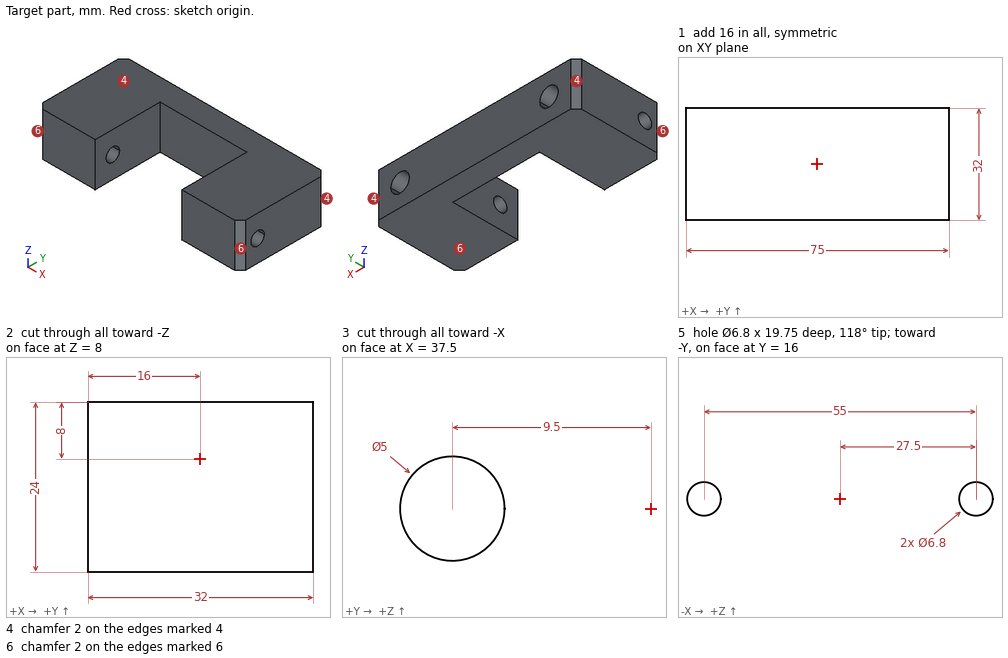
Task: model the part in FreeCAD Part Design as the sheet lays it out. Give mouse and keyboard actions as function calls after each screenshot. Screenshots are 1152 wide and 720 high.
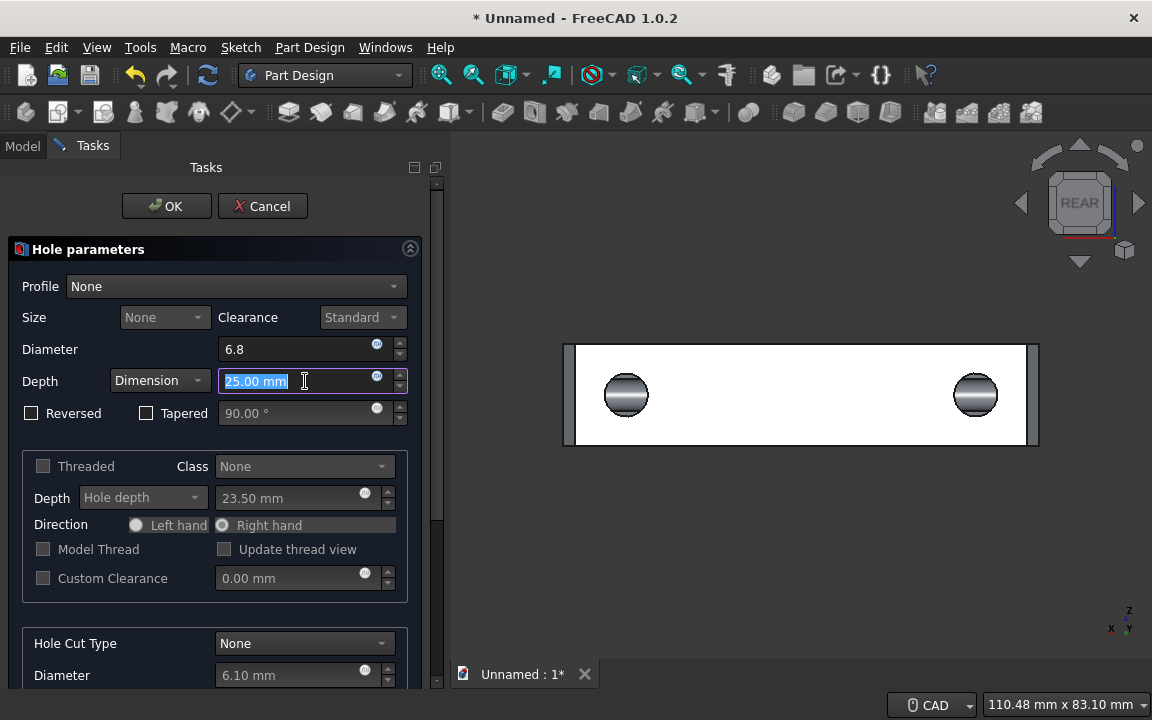
text(19.75)
key(Tab)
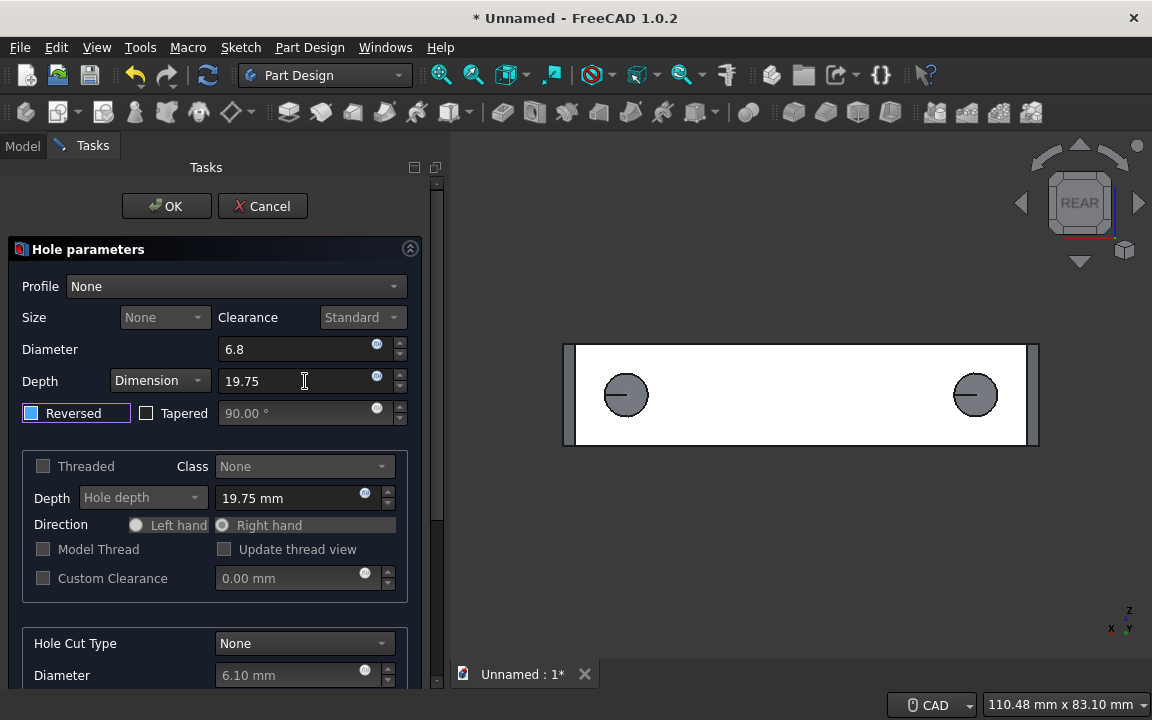
click(167, 206)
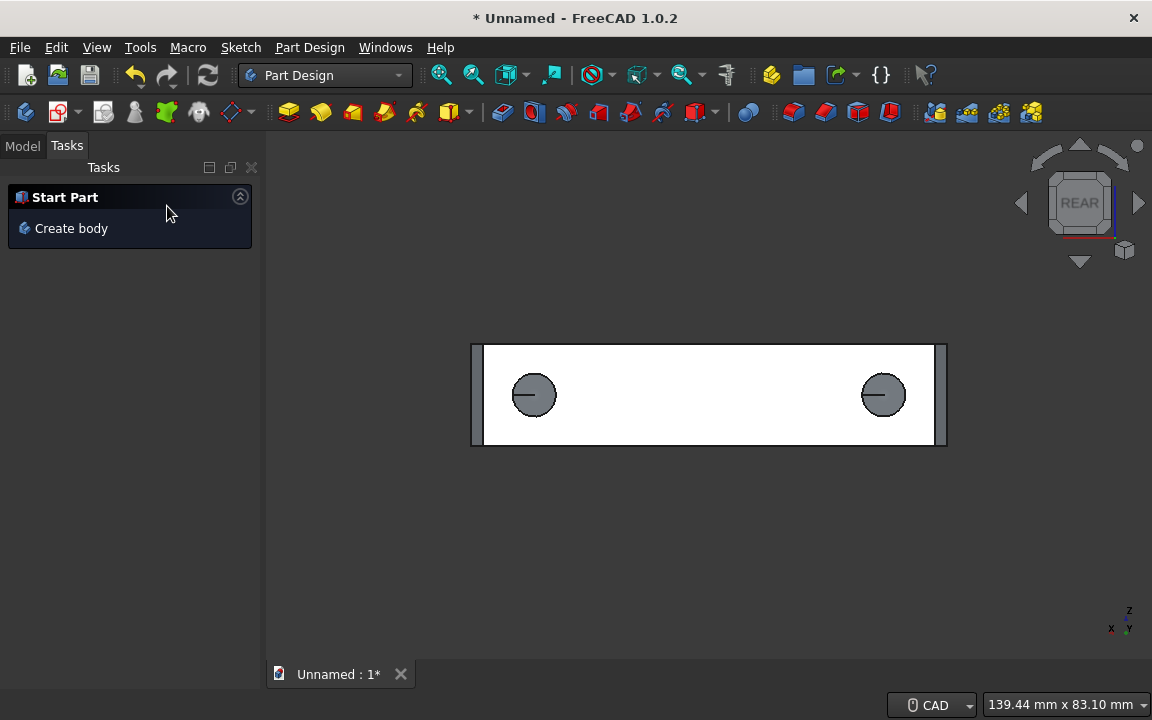
key(0)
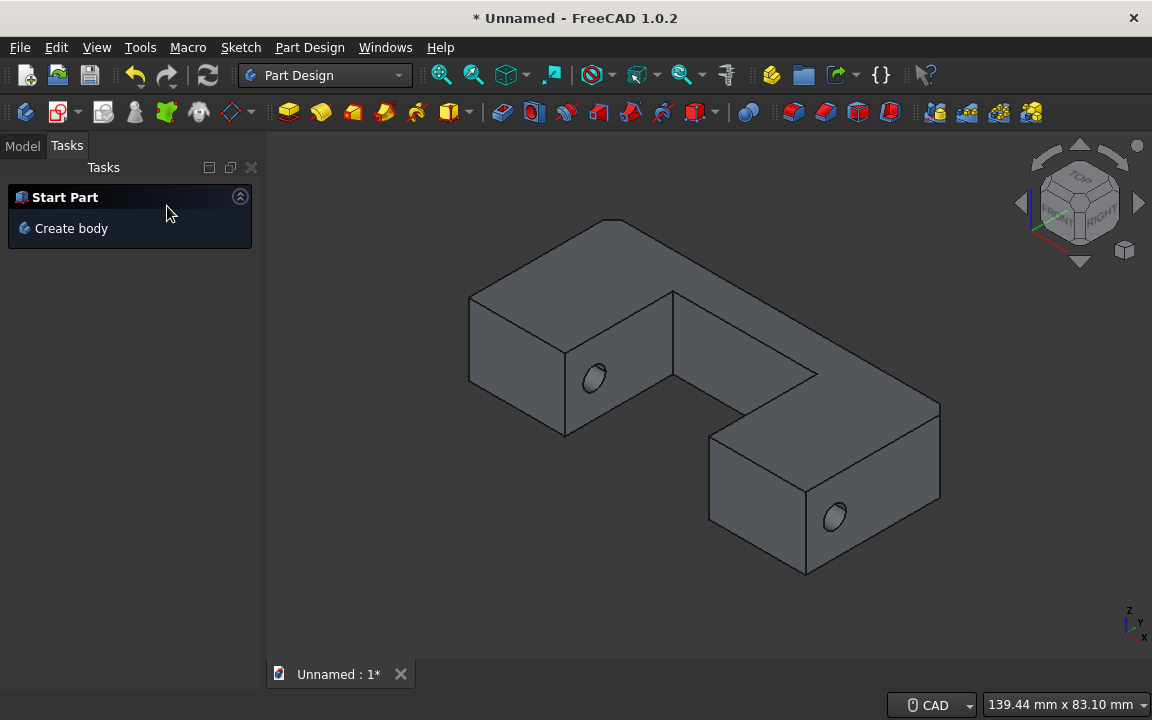
click(806, 533)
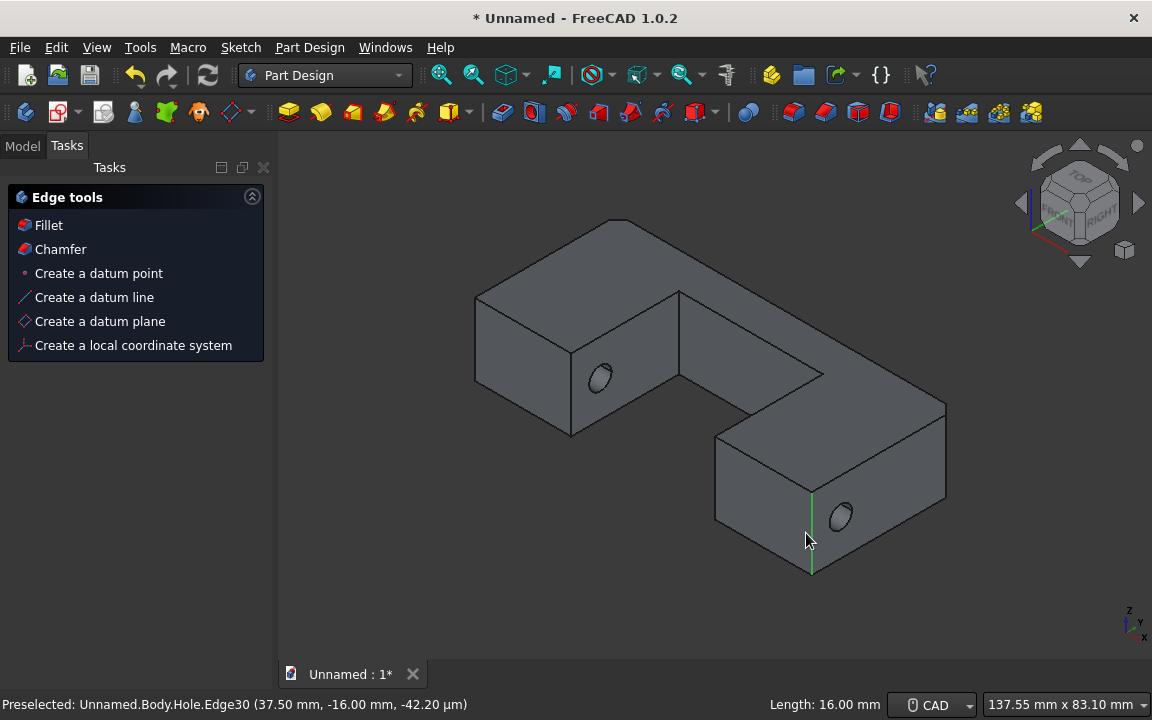
key(2)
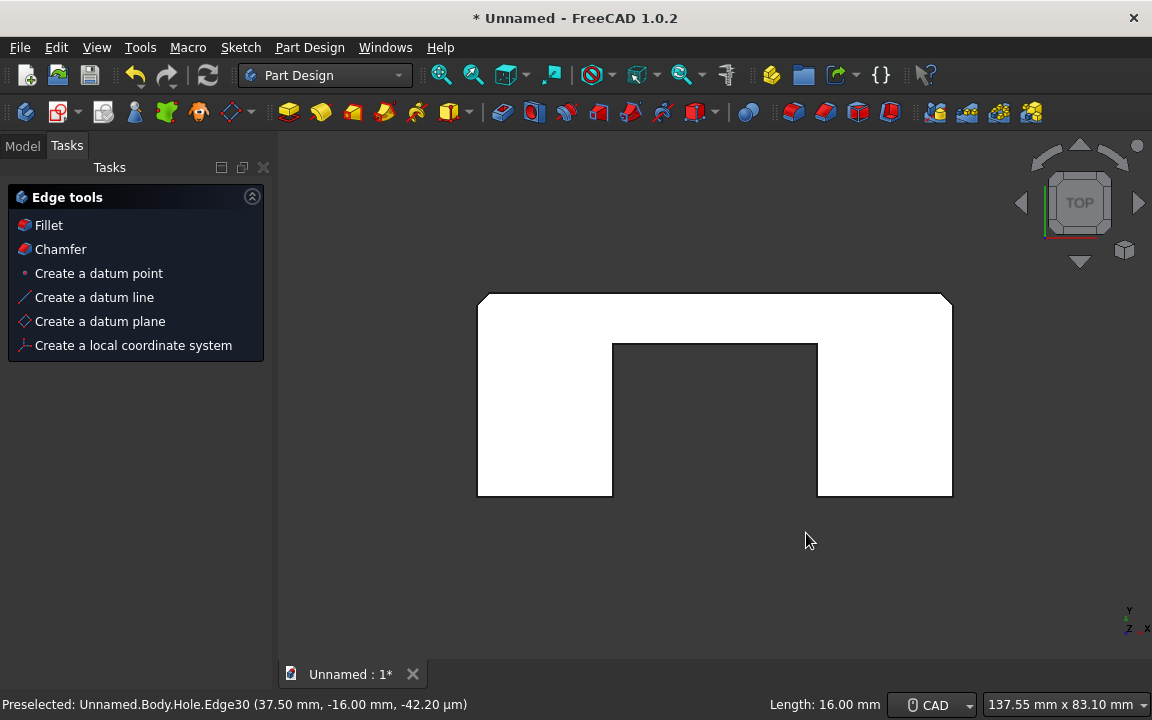
key(1)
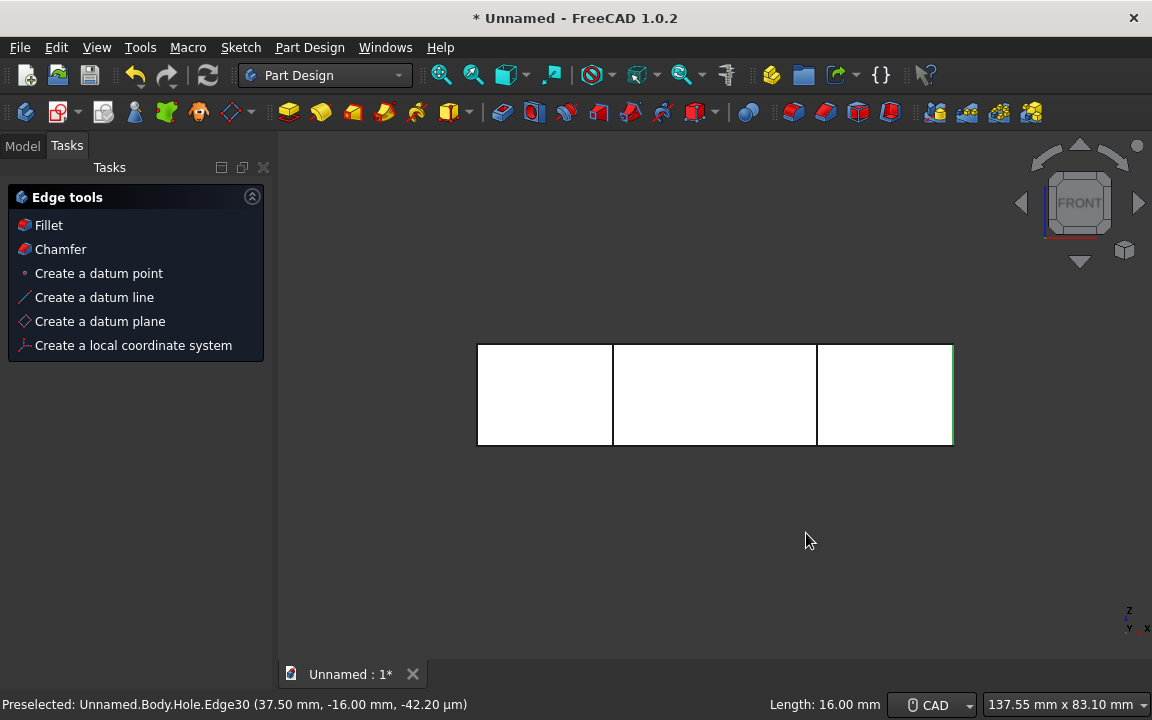
click(477, 394, ctrl)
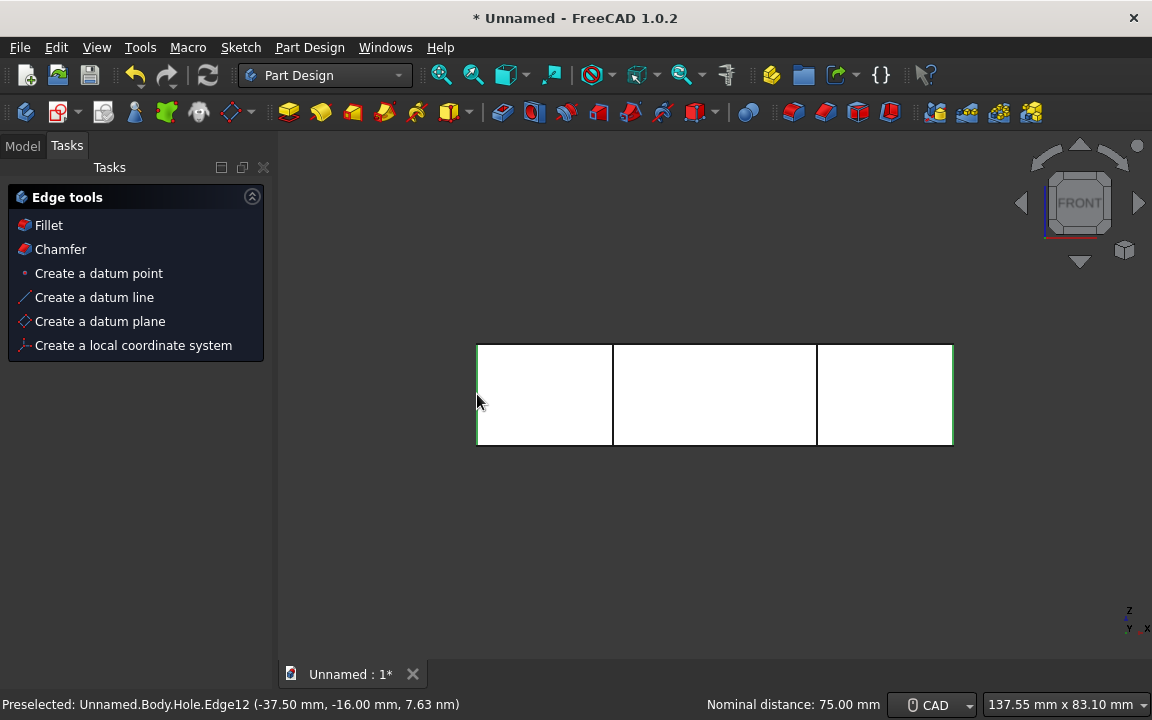
click(826, 112)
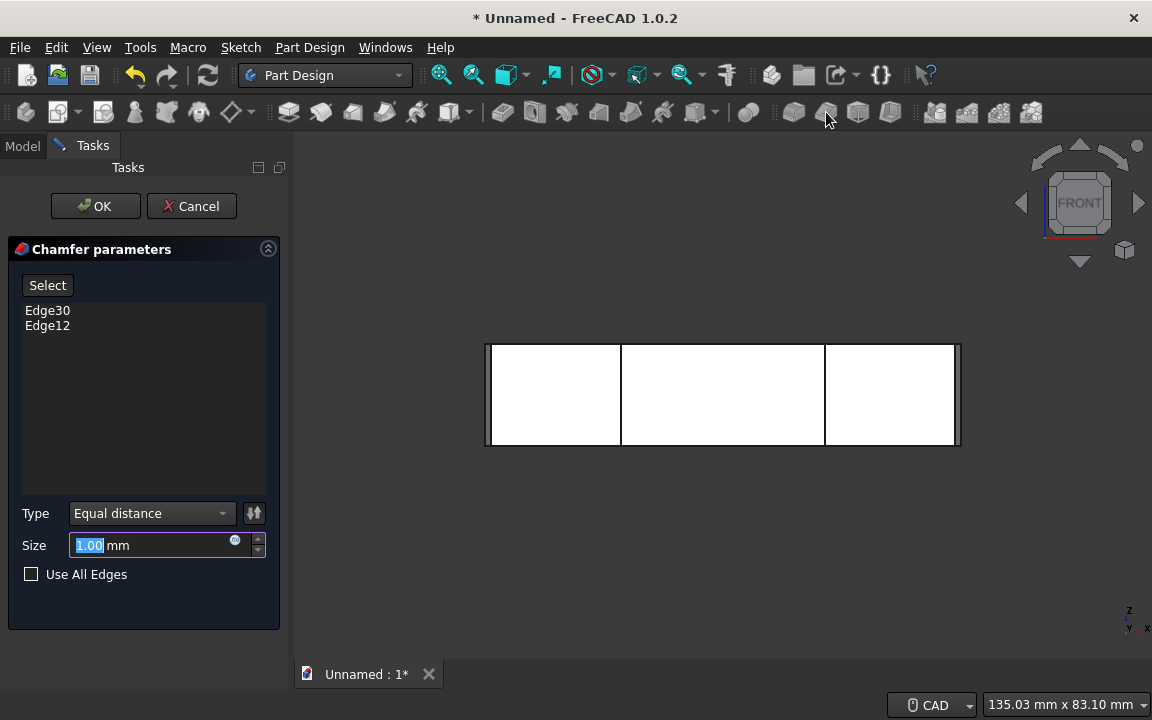
text(2)
key(Tab)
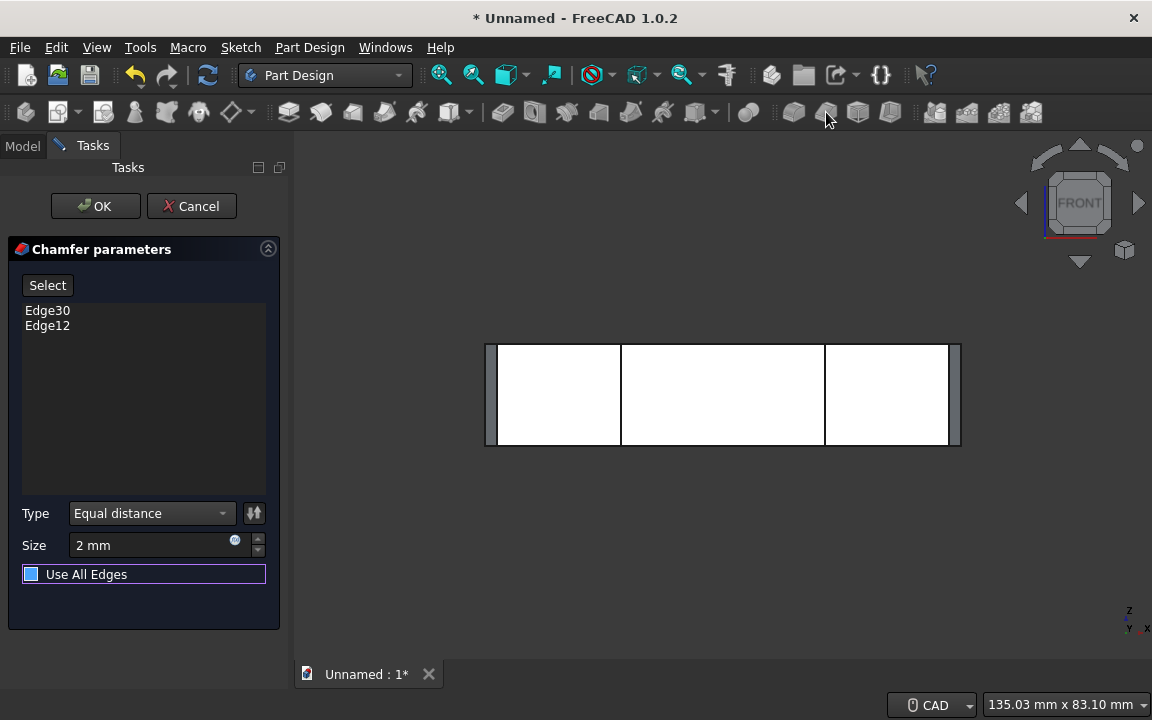
click(96, 206)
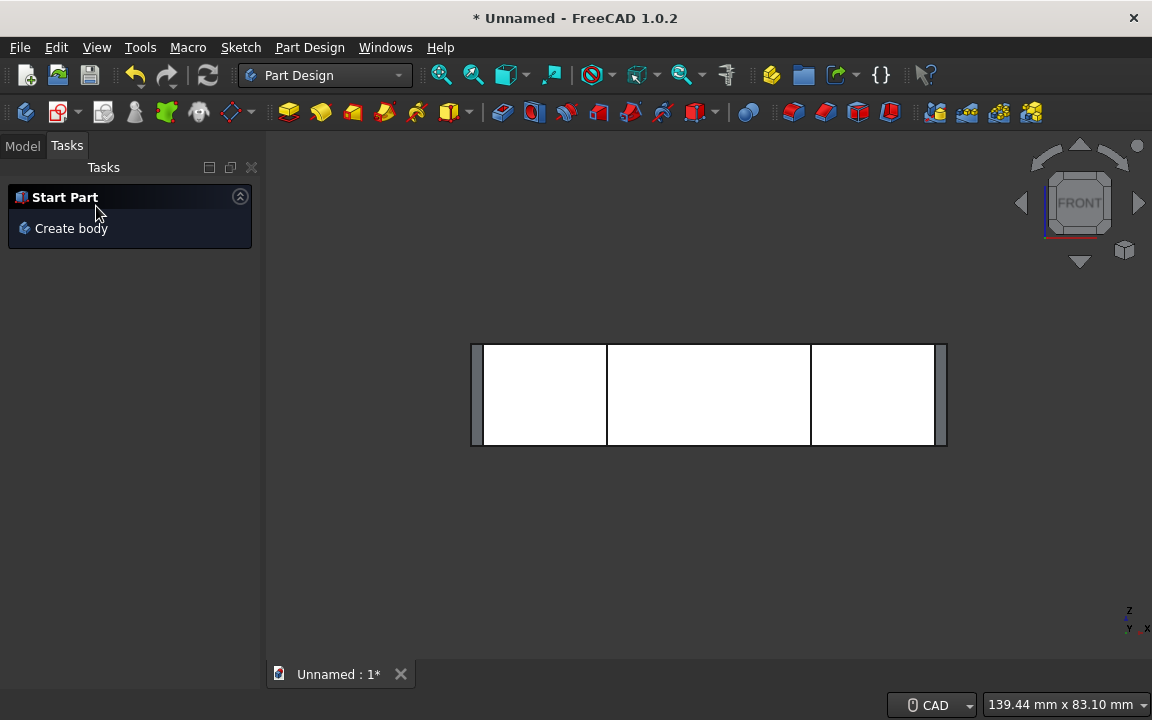
key(0)